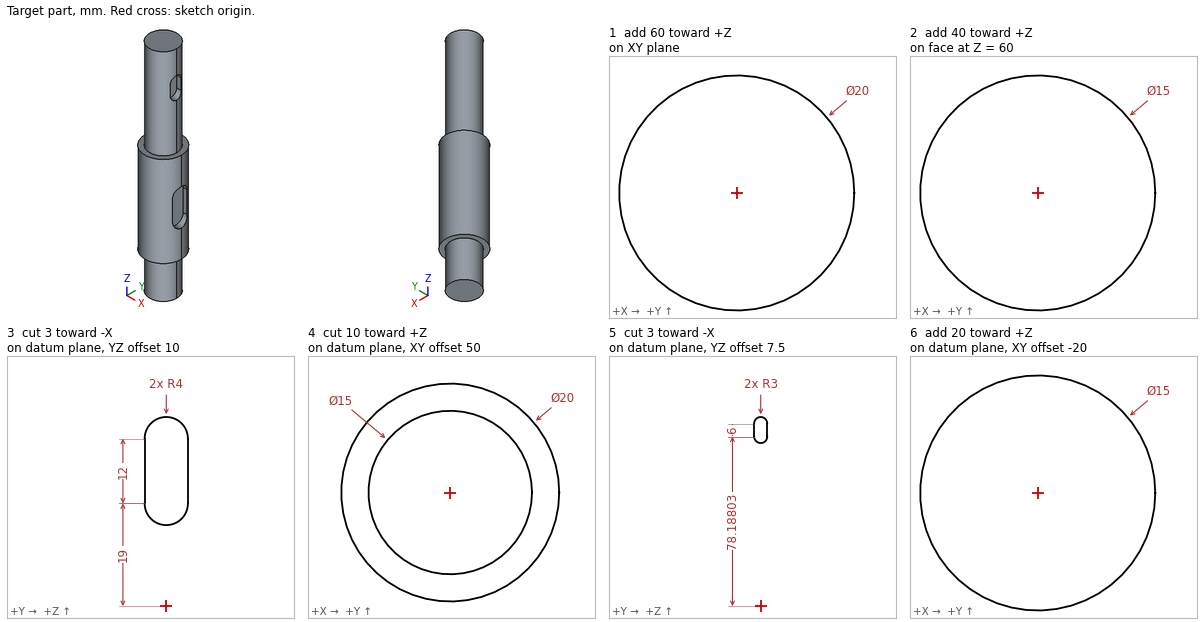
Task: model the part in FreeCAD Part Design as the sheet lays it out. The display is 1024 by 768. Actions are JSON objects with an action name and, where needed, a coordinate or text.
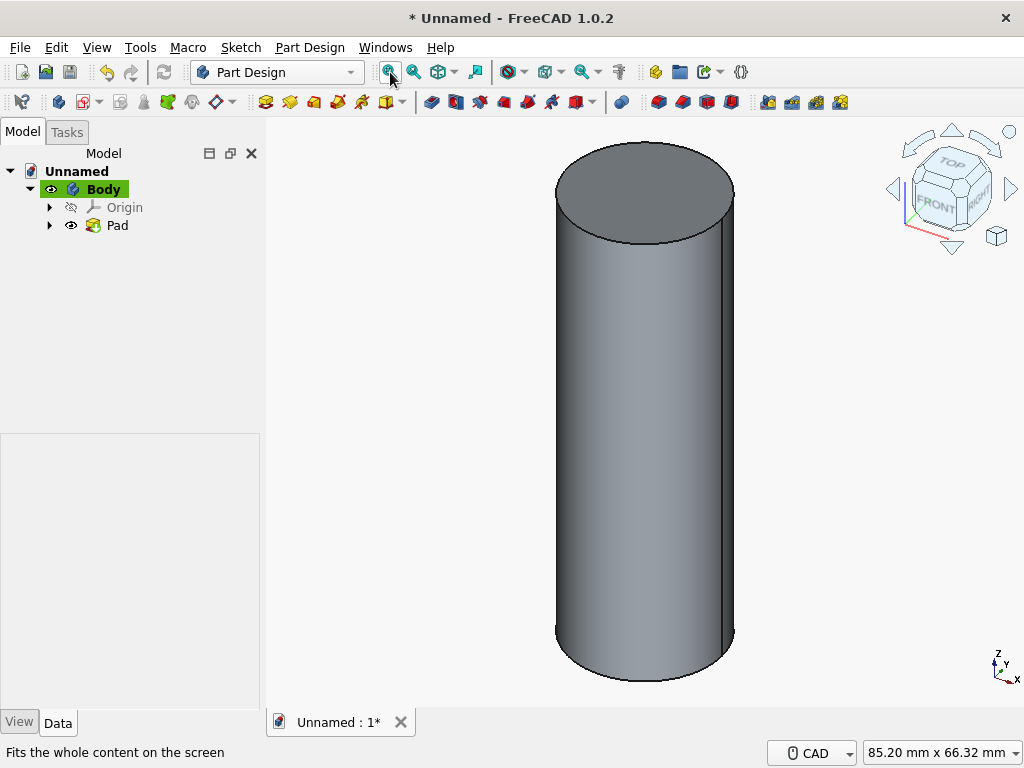
{"action": "left_click", "coordinate": [645, 192]}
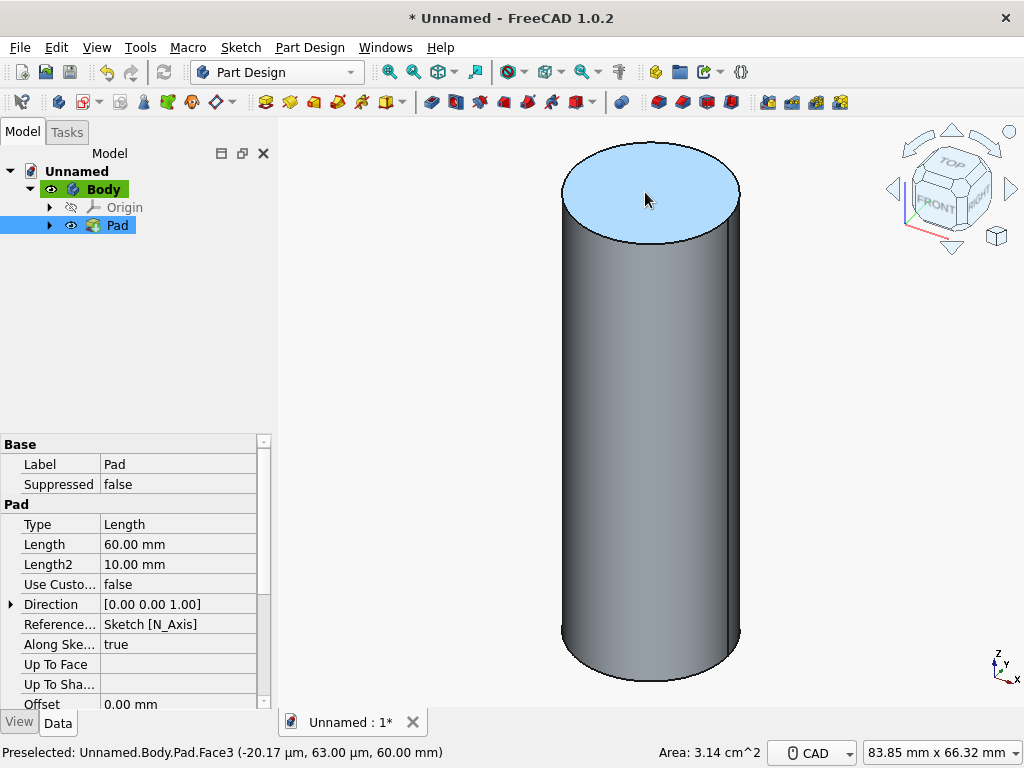
{"action": "left_click", "coordinate": [84, 102]}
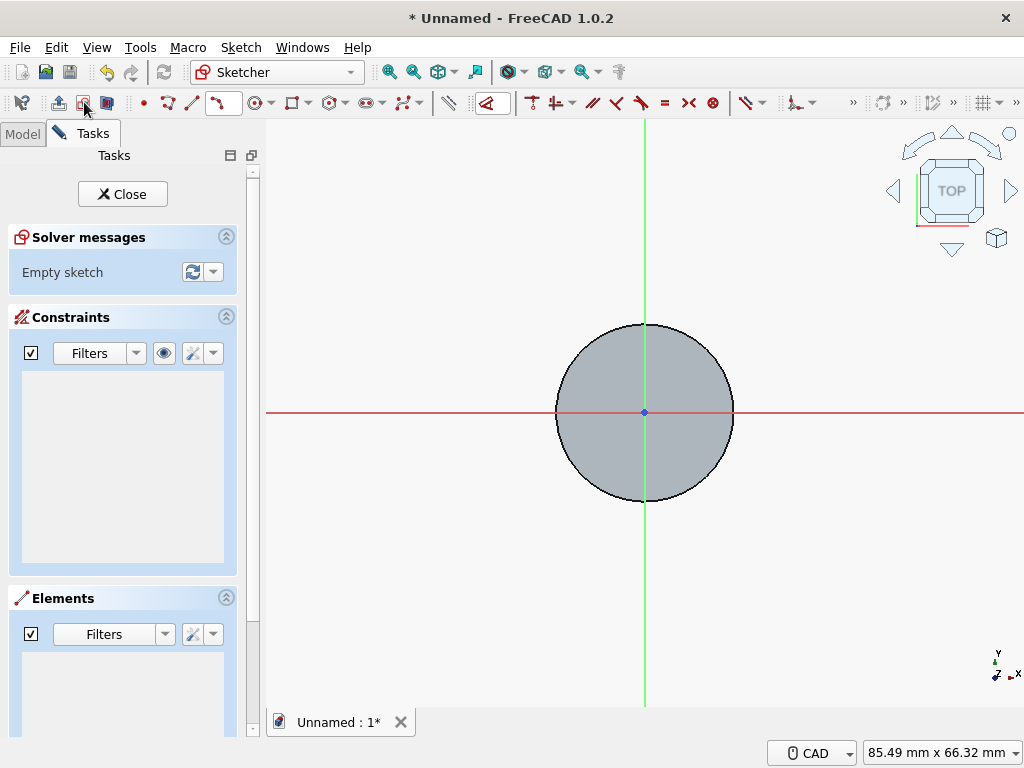
{"action": "scroll", "coordinate": [685, 413], "scroll_direction": "up", "scroll_amount": 5}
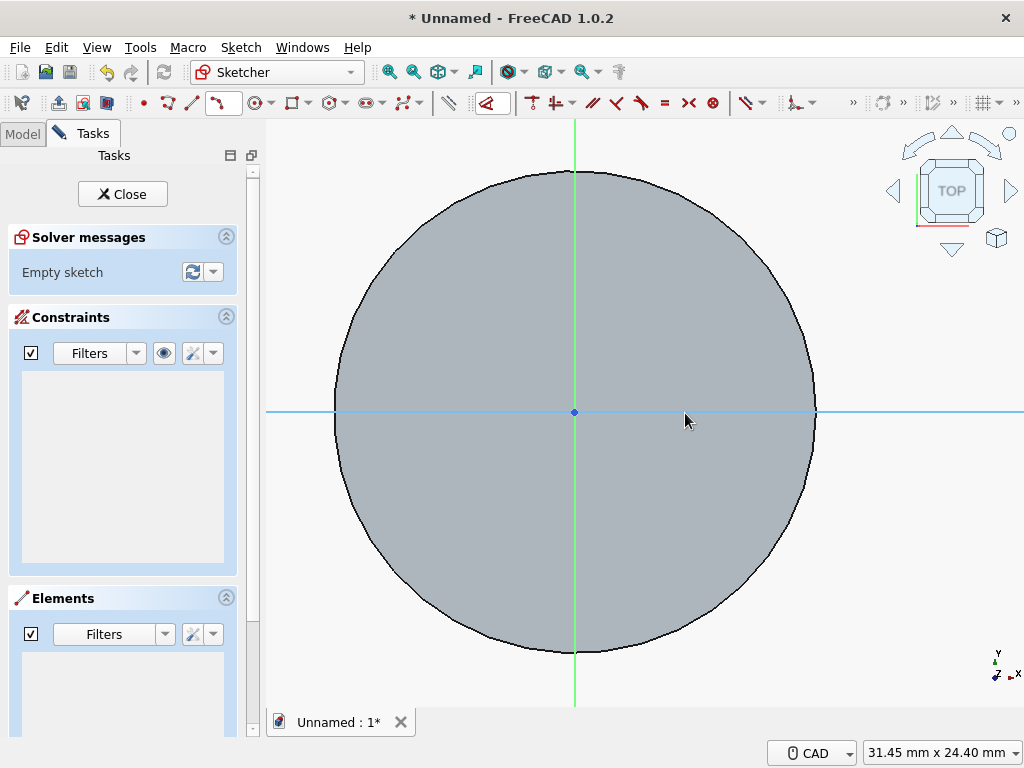
{"action": "left_click", "coordinate": [256, 104]}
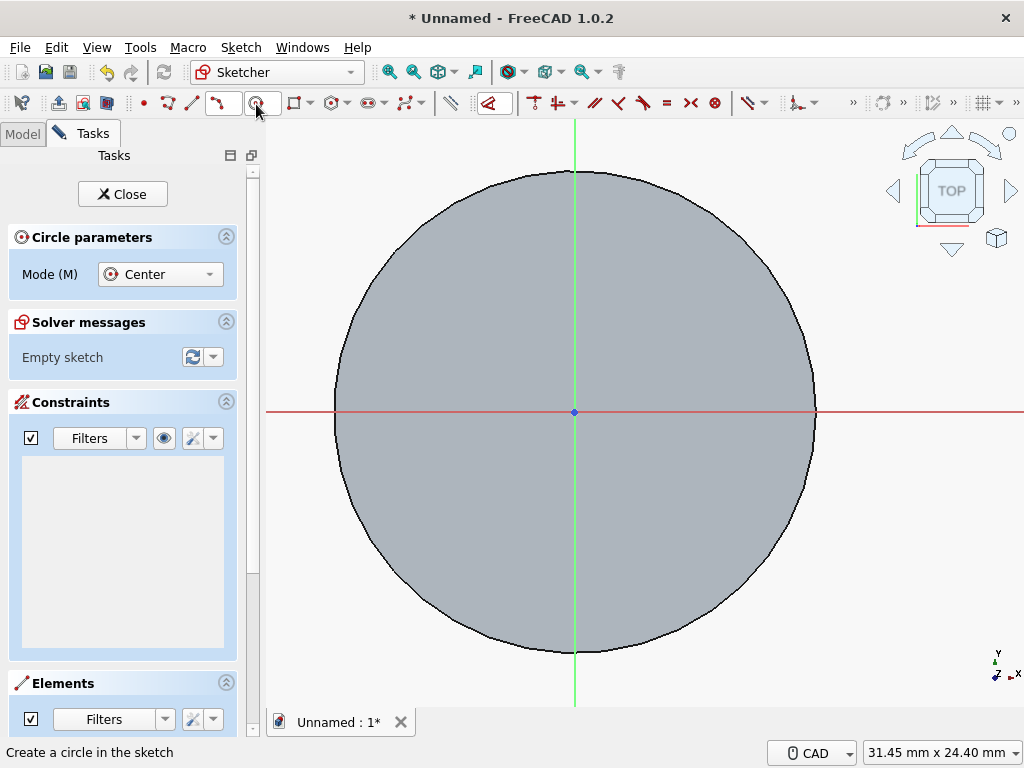
{"action": "left_click", "coordinate": [575, 412]}
{"action": "mouse_move", "coordinate": [703, 284]}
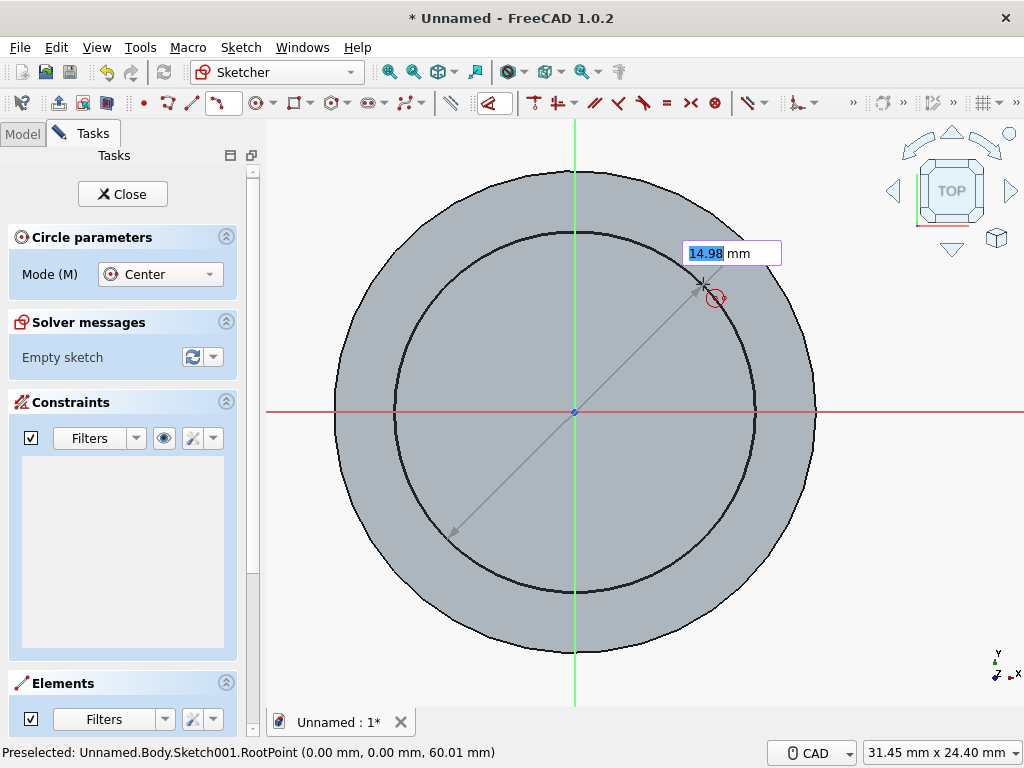
{"action": "type", "text": "15"}
{"action": "key", "text": "Return"}
{"action": "key", "text": "Escape"}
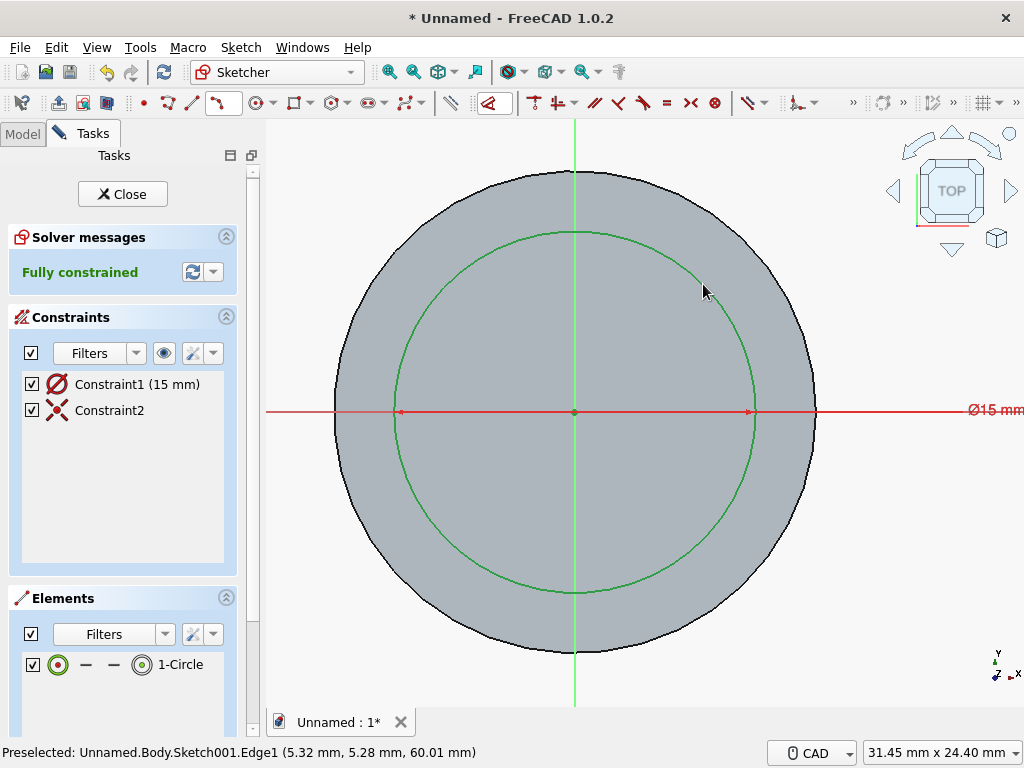
{"action": "left_click", "coordinate": [123, 194]}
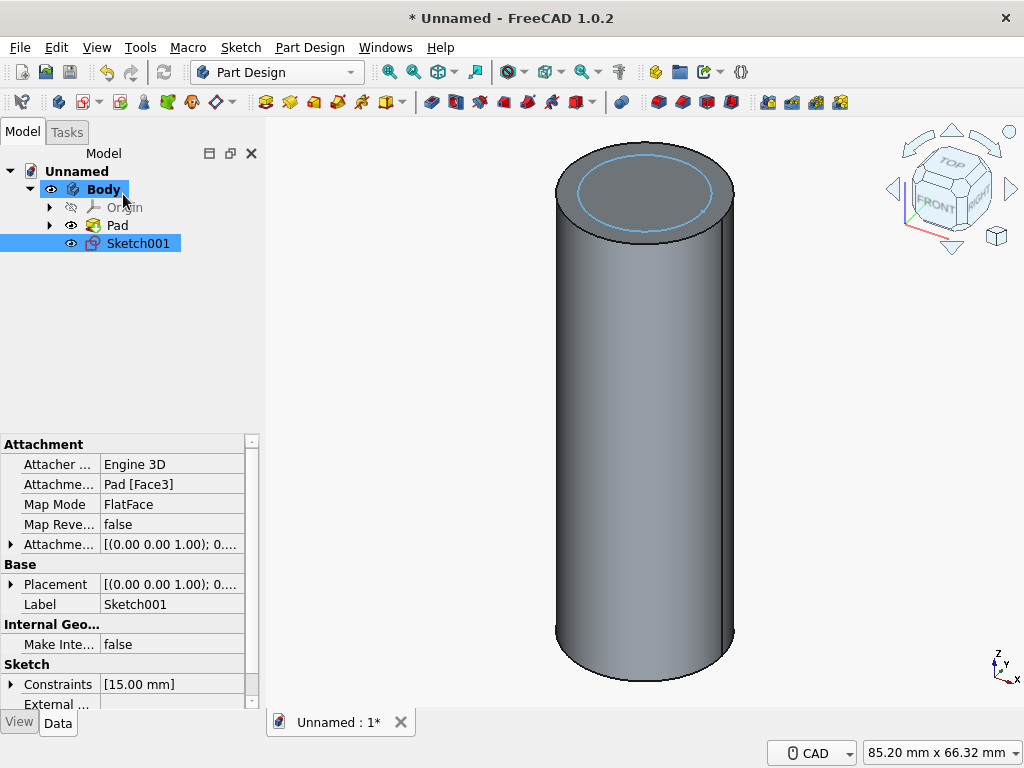
{"action": "left_click", "coordinate": [266, 102]}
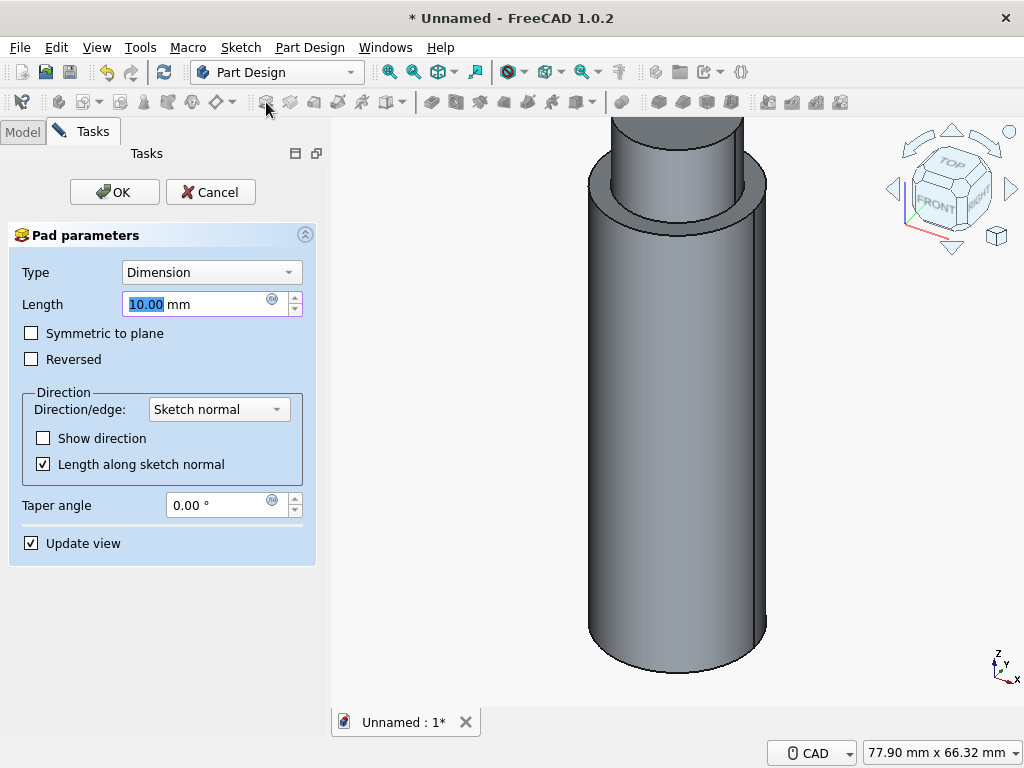
{"action": "type", "text": "40"}
{"action": "key", "text": "Tab"}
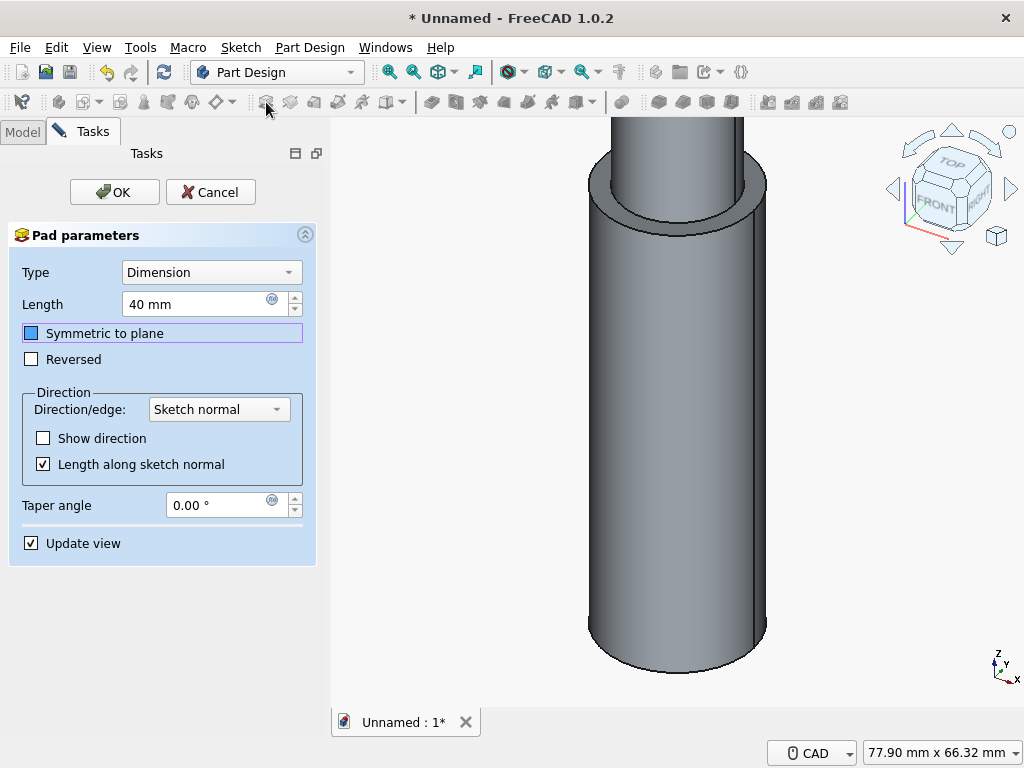
{"action": "left_click", "coordinate": [115, 192]}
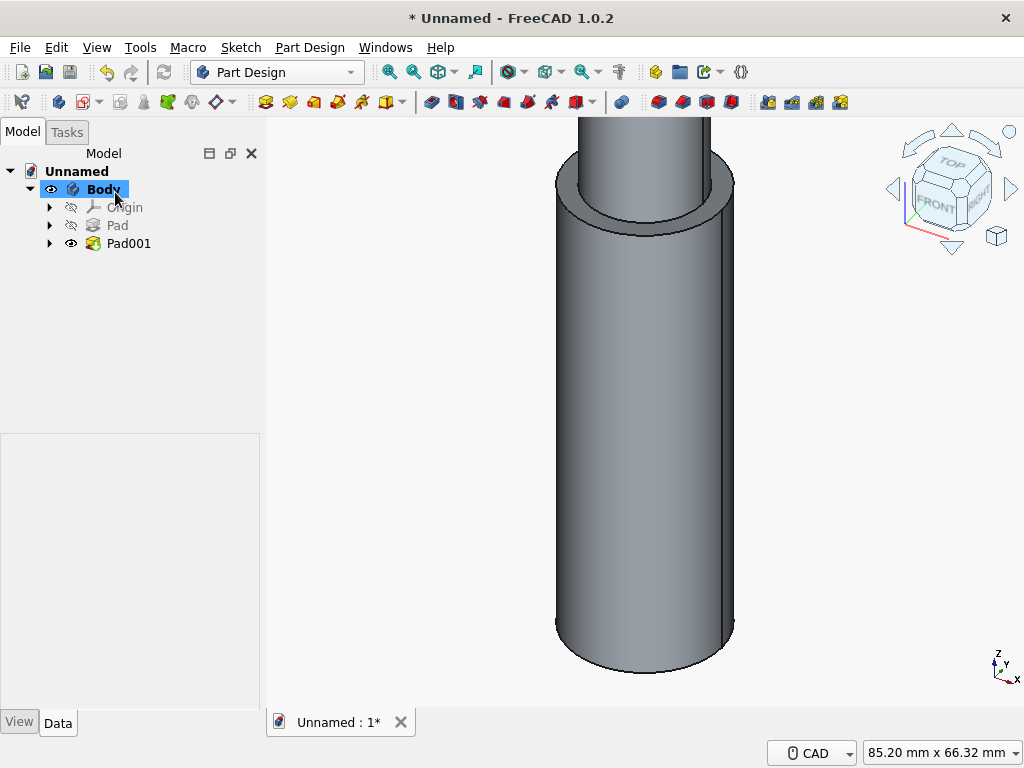
{"action": "left_click", "coordinate": [390, 72]}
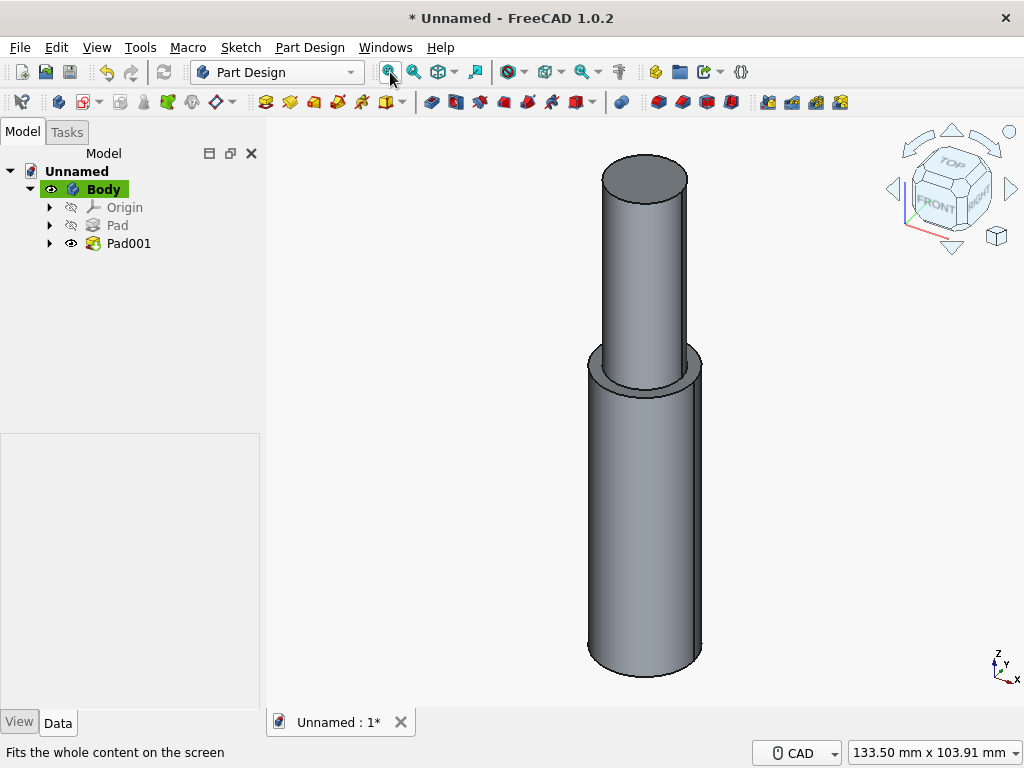
{"action": "left_click", "coordinate": [50, 207]}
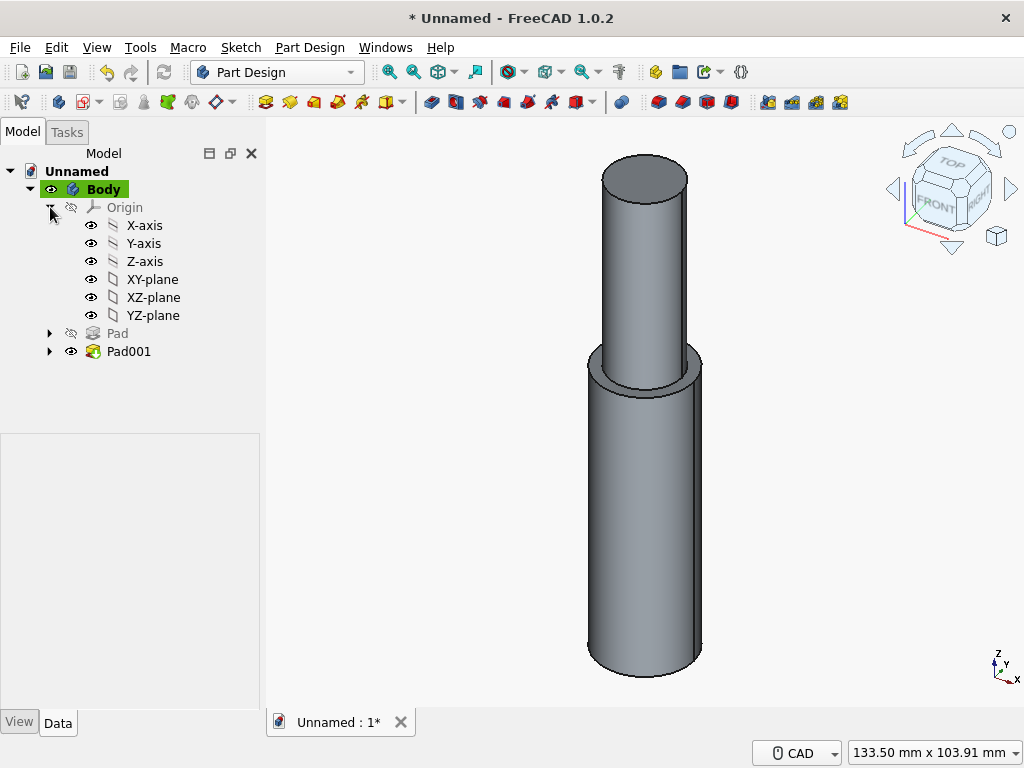
{"action": "left_click", "coordinate": [136, 315]}